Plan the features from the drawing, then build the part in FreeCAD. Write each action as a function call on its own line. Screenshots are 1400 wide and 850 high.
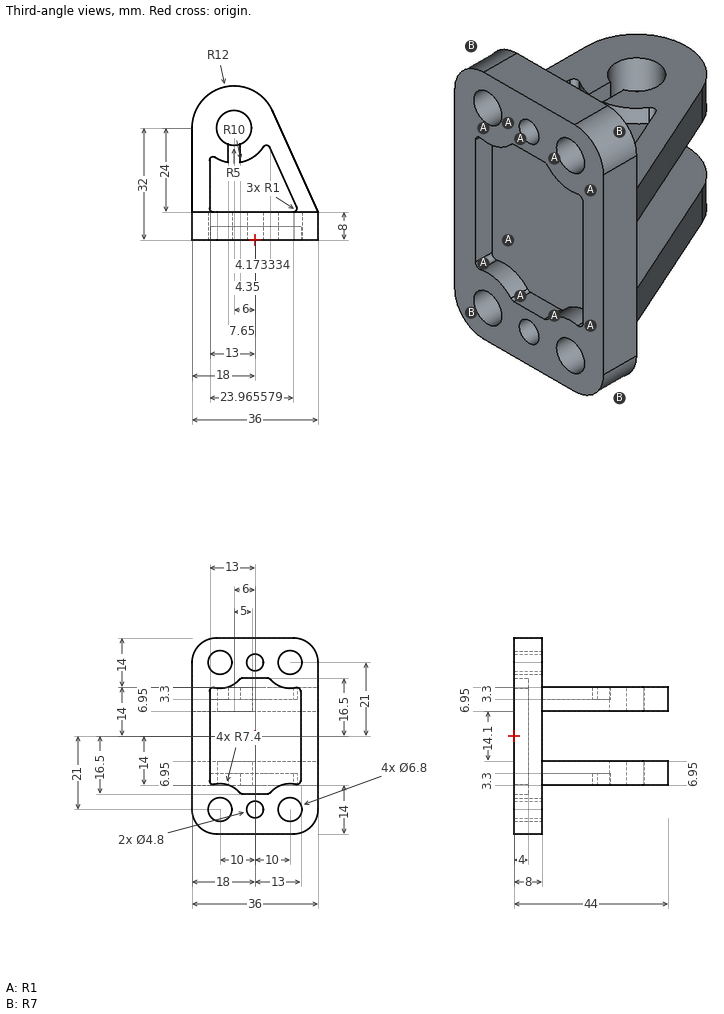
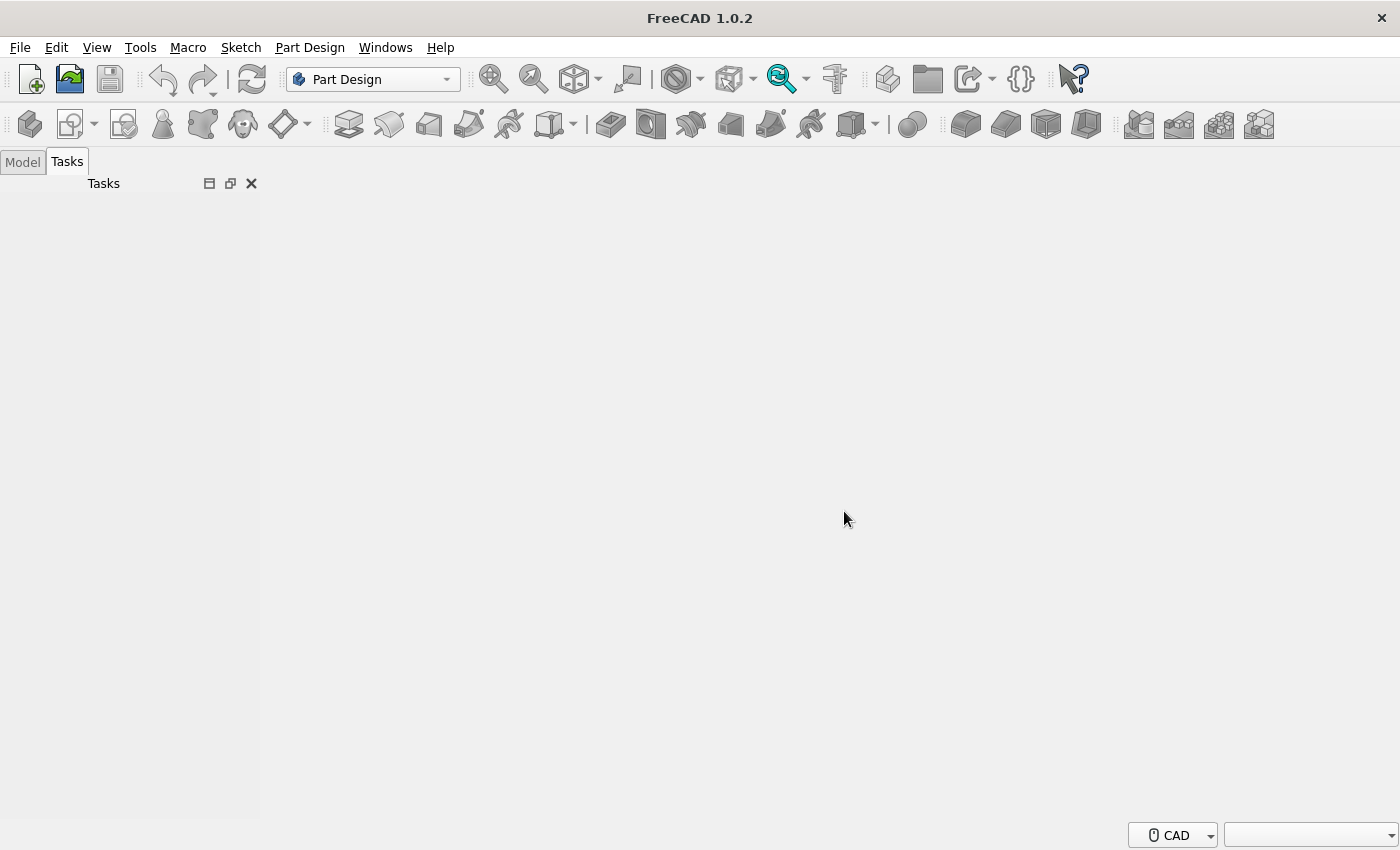
key(ctrl+n)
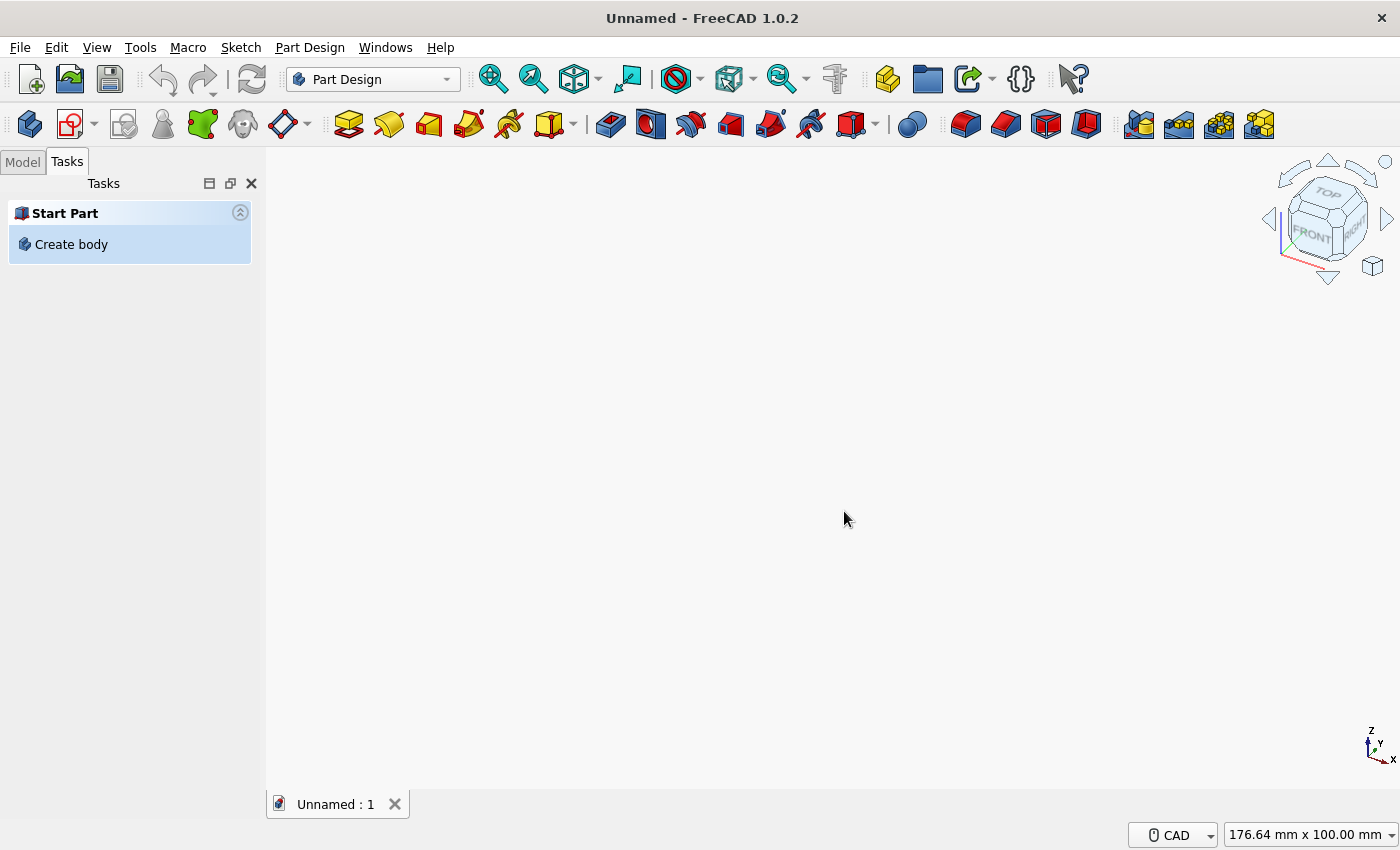
click(30, 124)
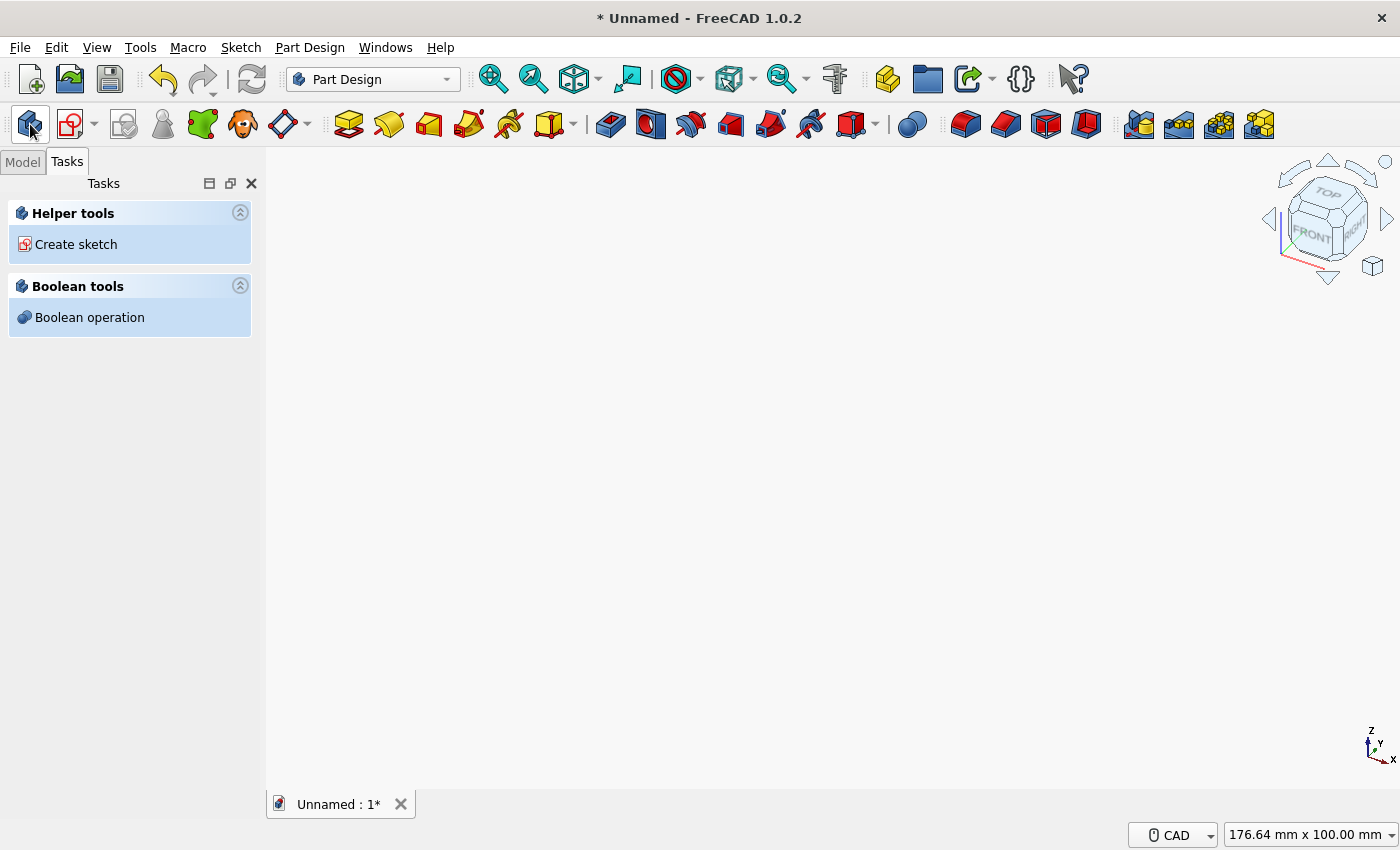
click(23, 161)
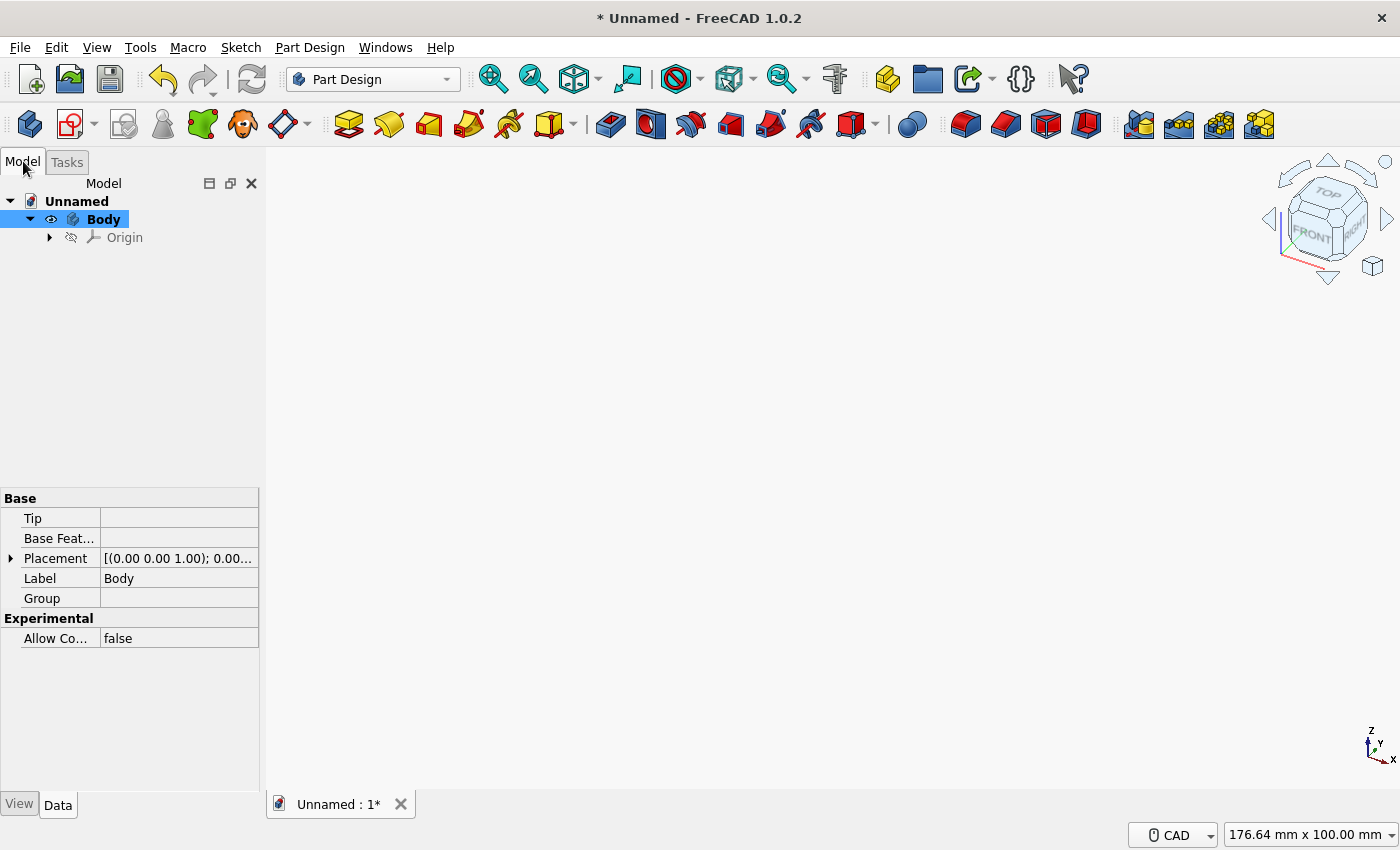
click(50, 237)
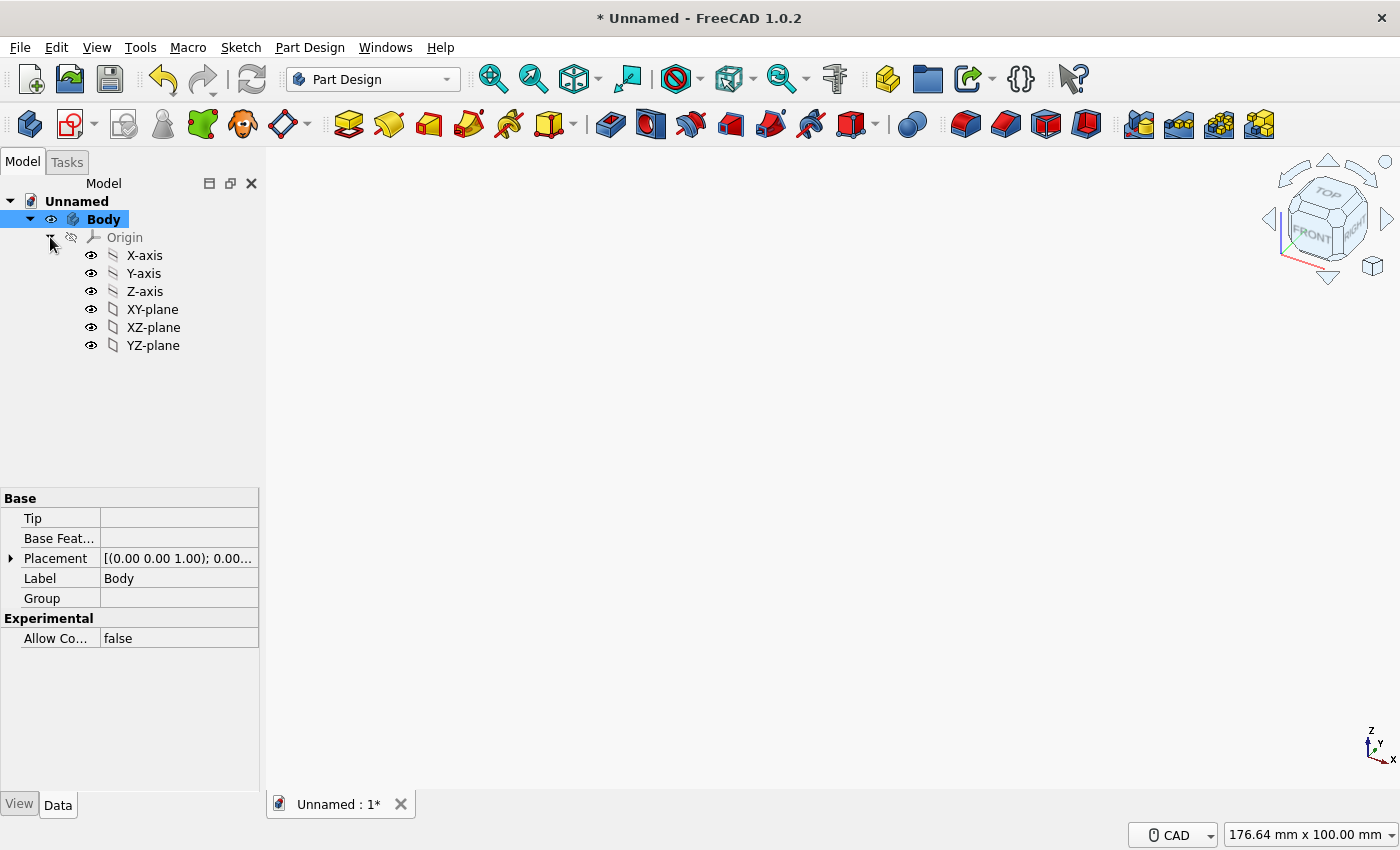
click(136, 309)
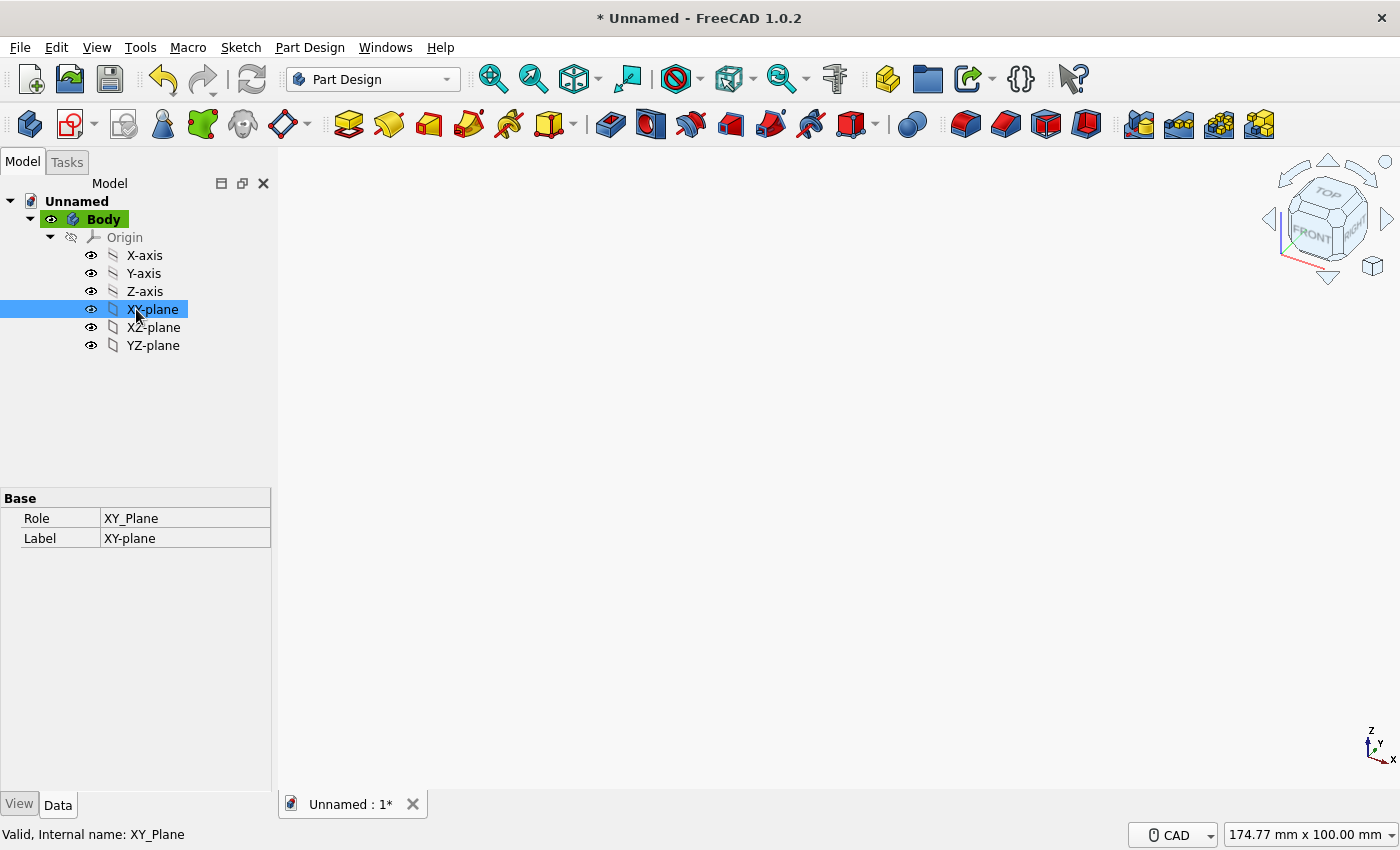
click(284, 124)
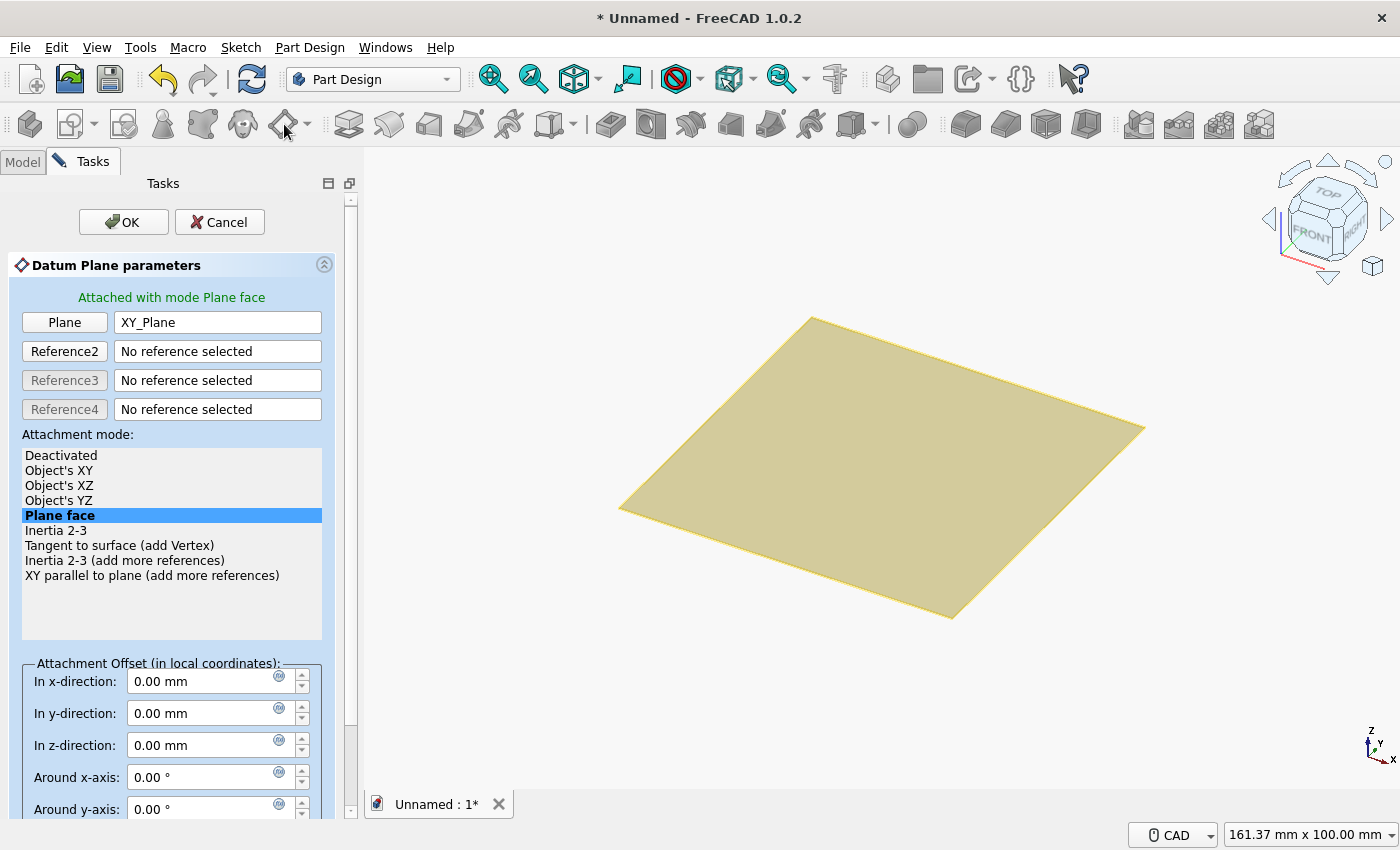
triple_click(210, 745)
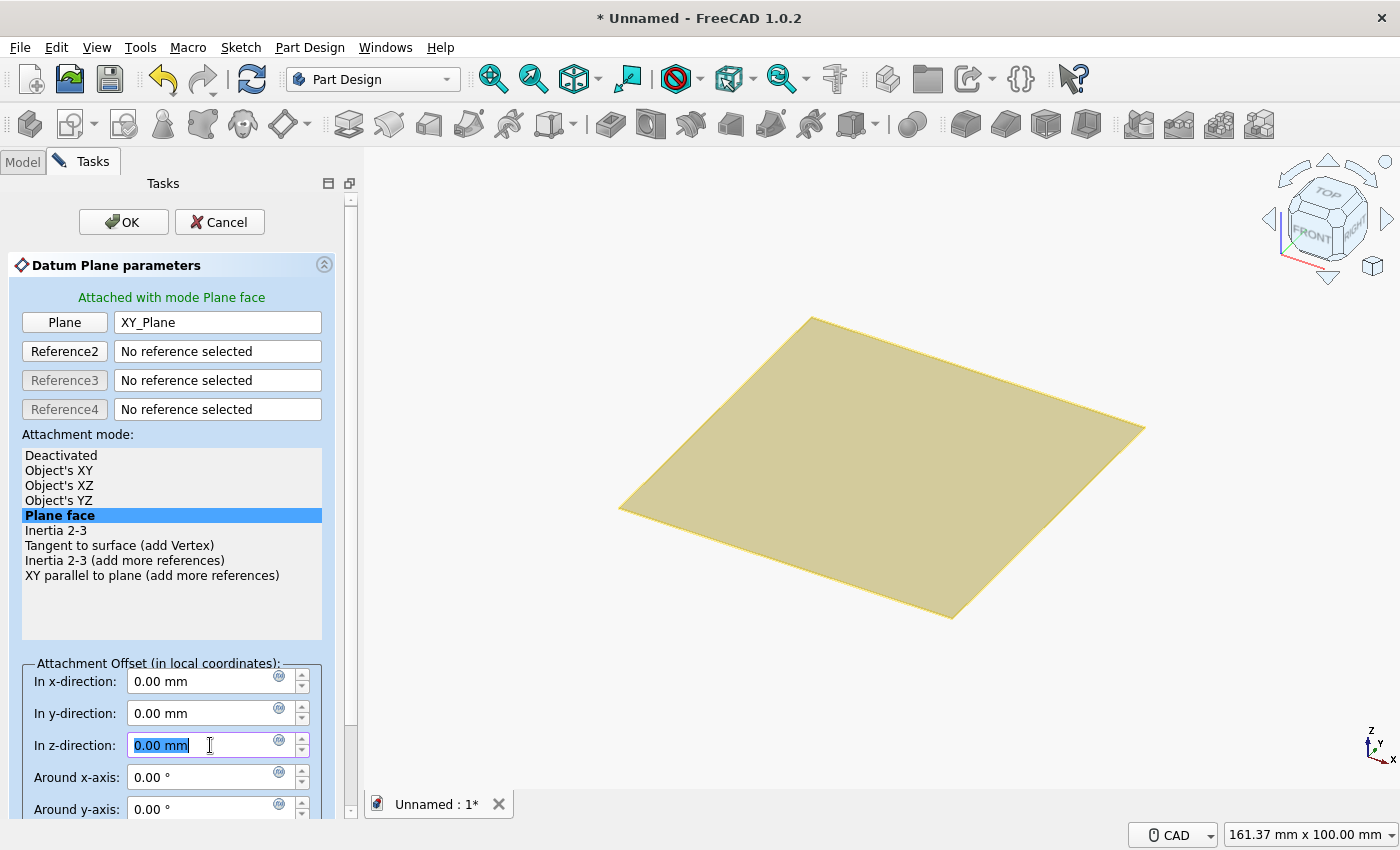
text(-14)
key(Tab)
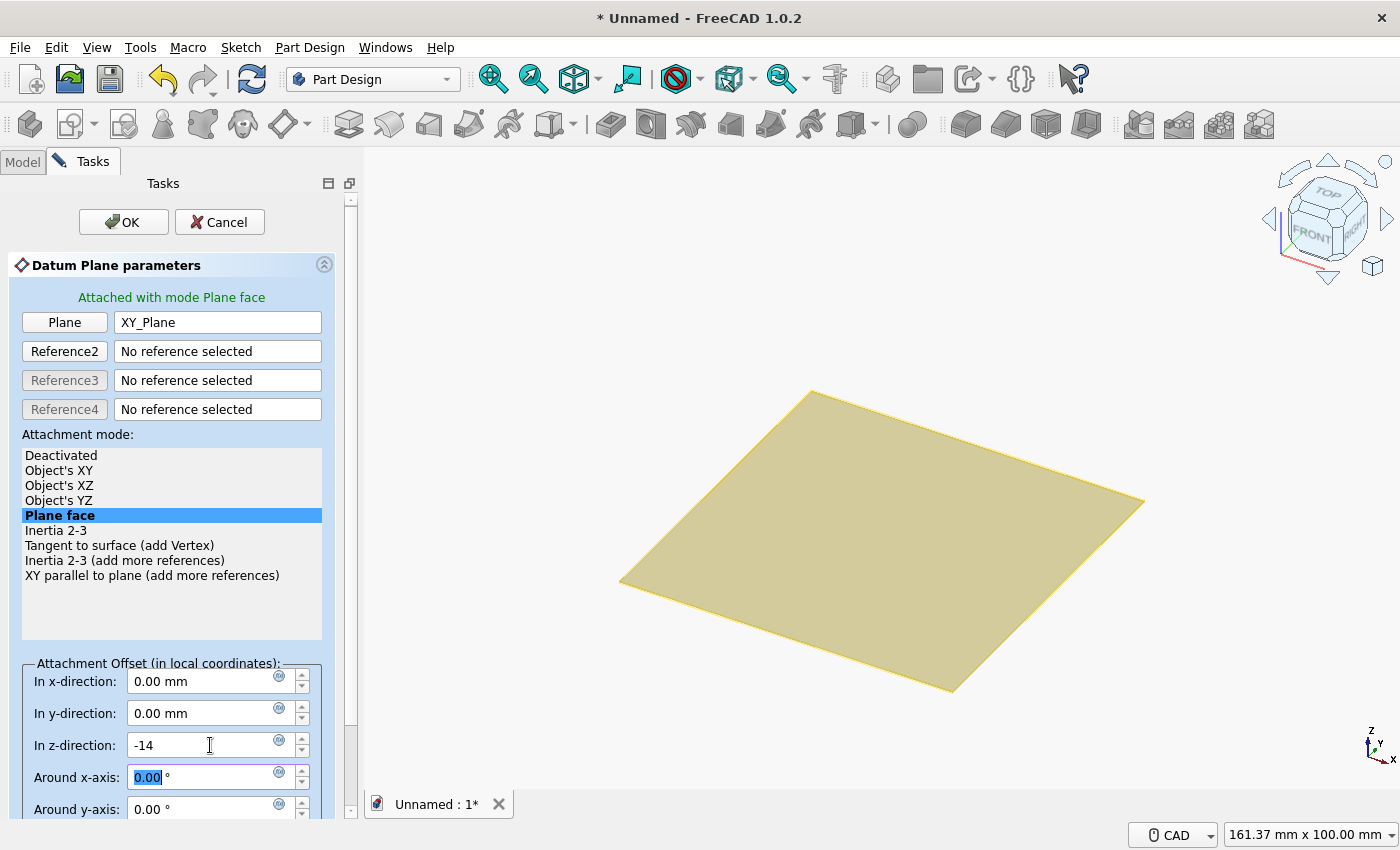
click(124, 222)